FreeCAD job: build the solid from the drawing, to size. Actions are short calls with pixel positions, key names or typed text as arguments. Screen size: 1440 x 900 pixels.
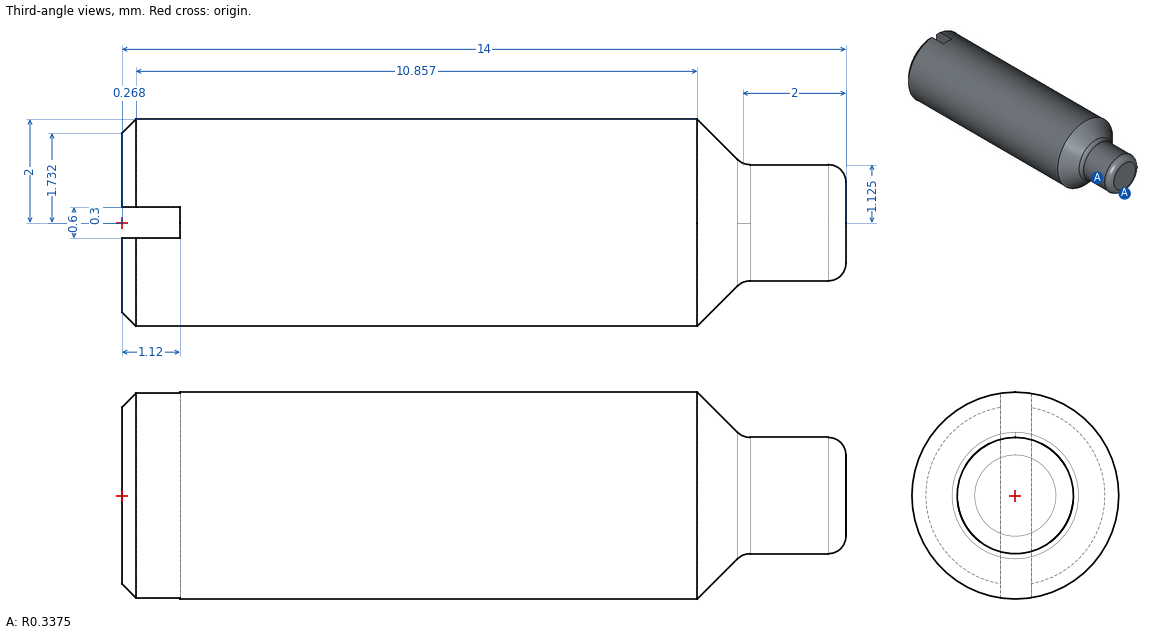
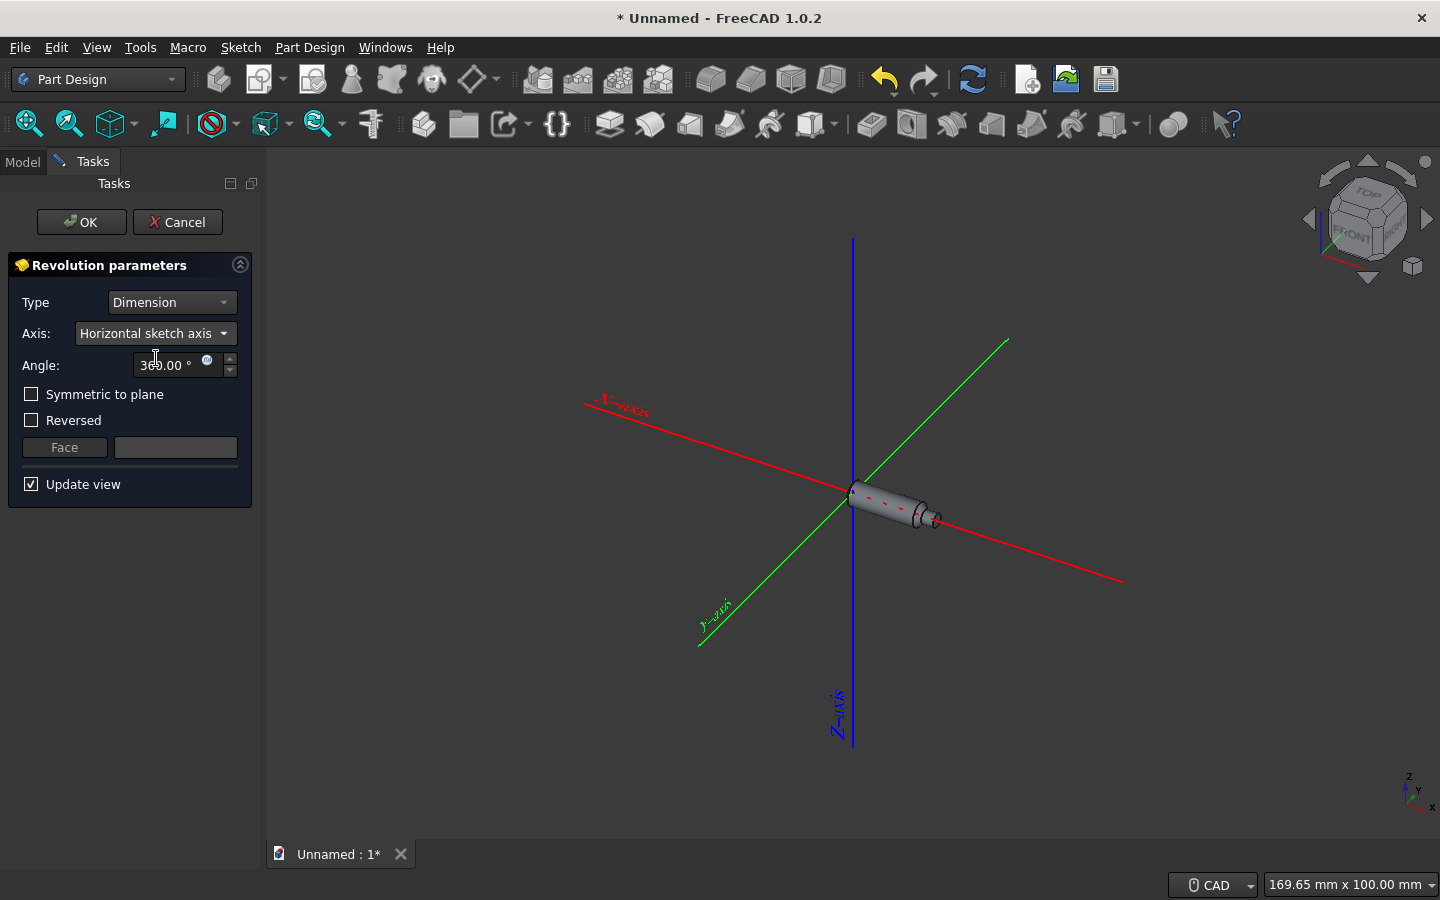
click(82, 222)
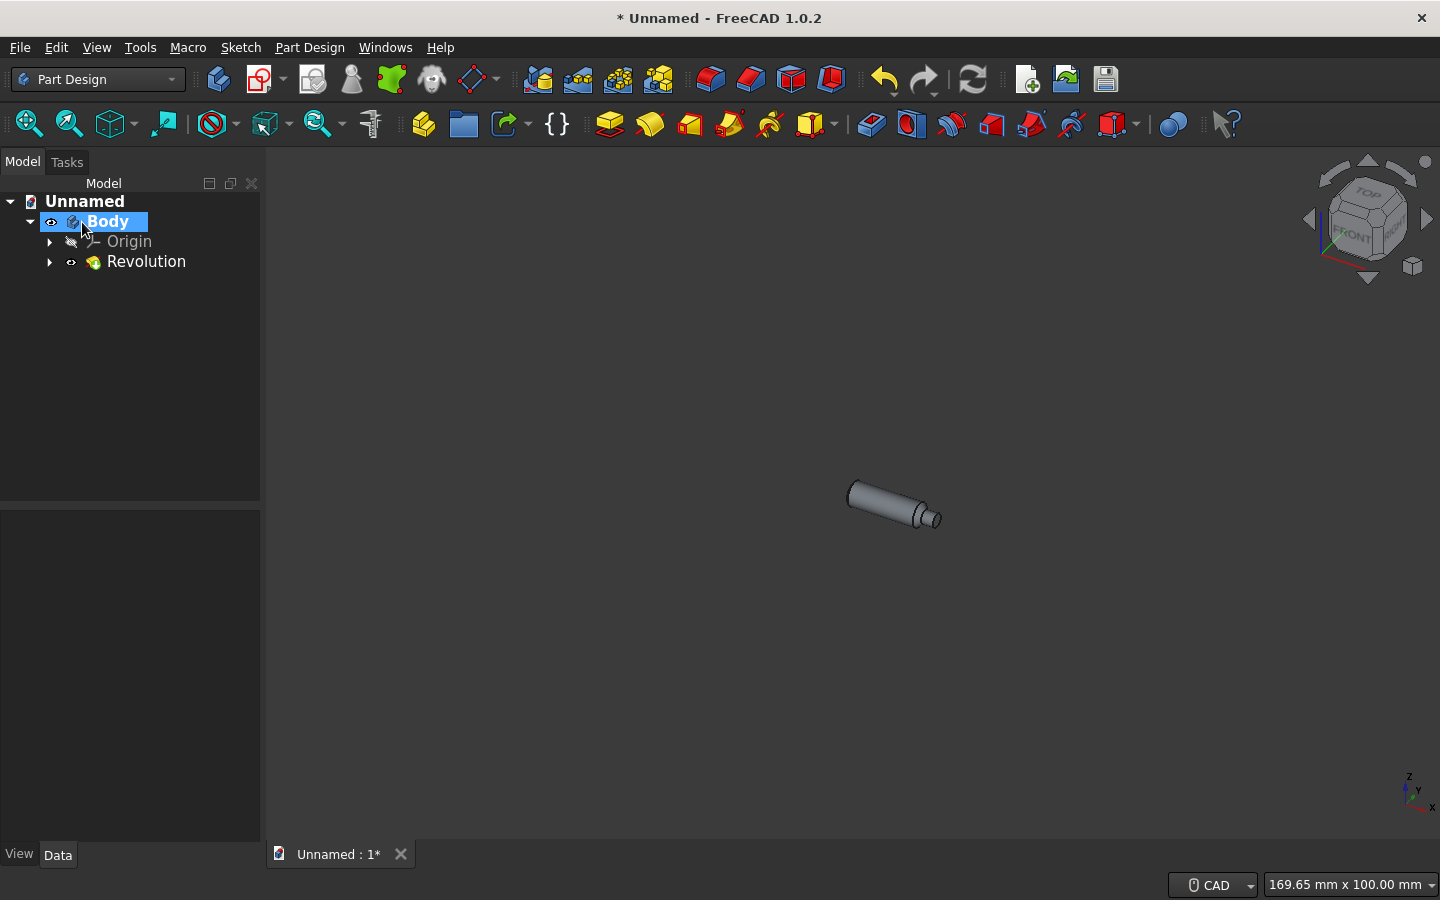
key(v)
key(f)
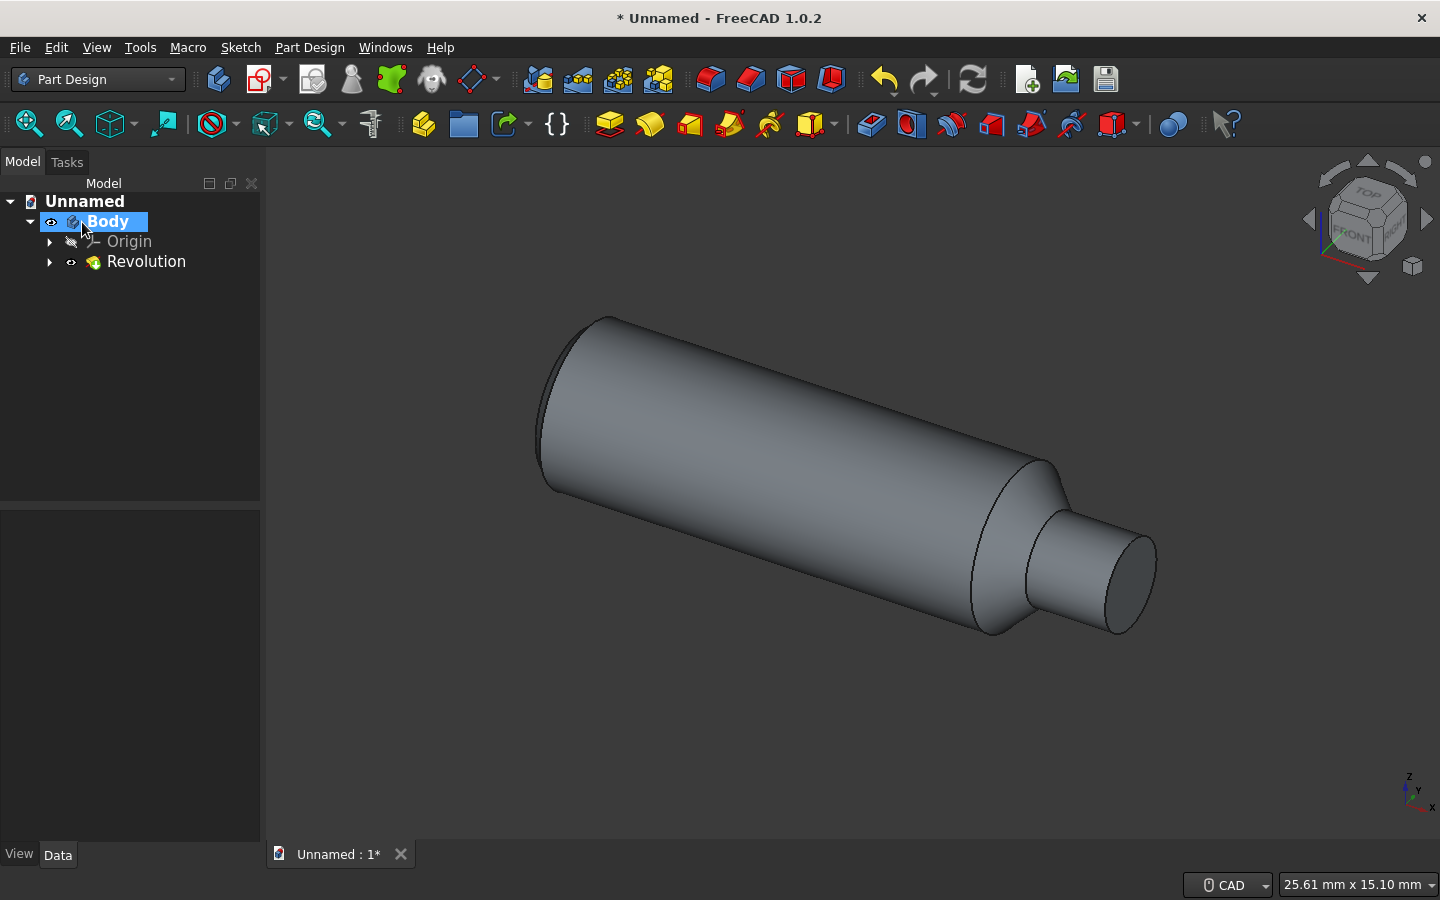
click(260, 80)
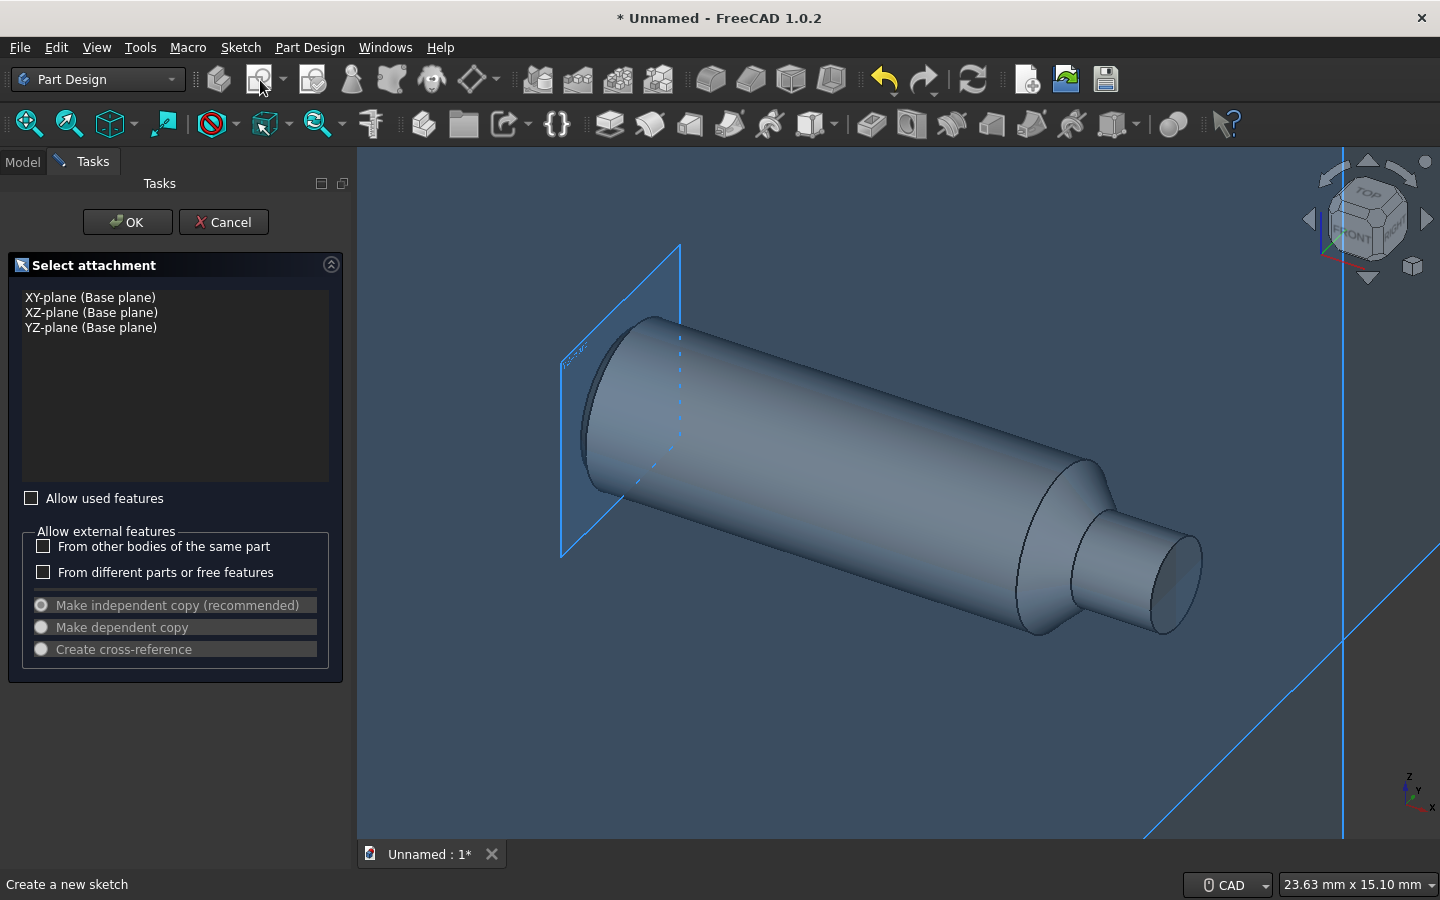
click(82, 298)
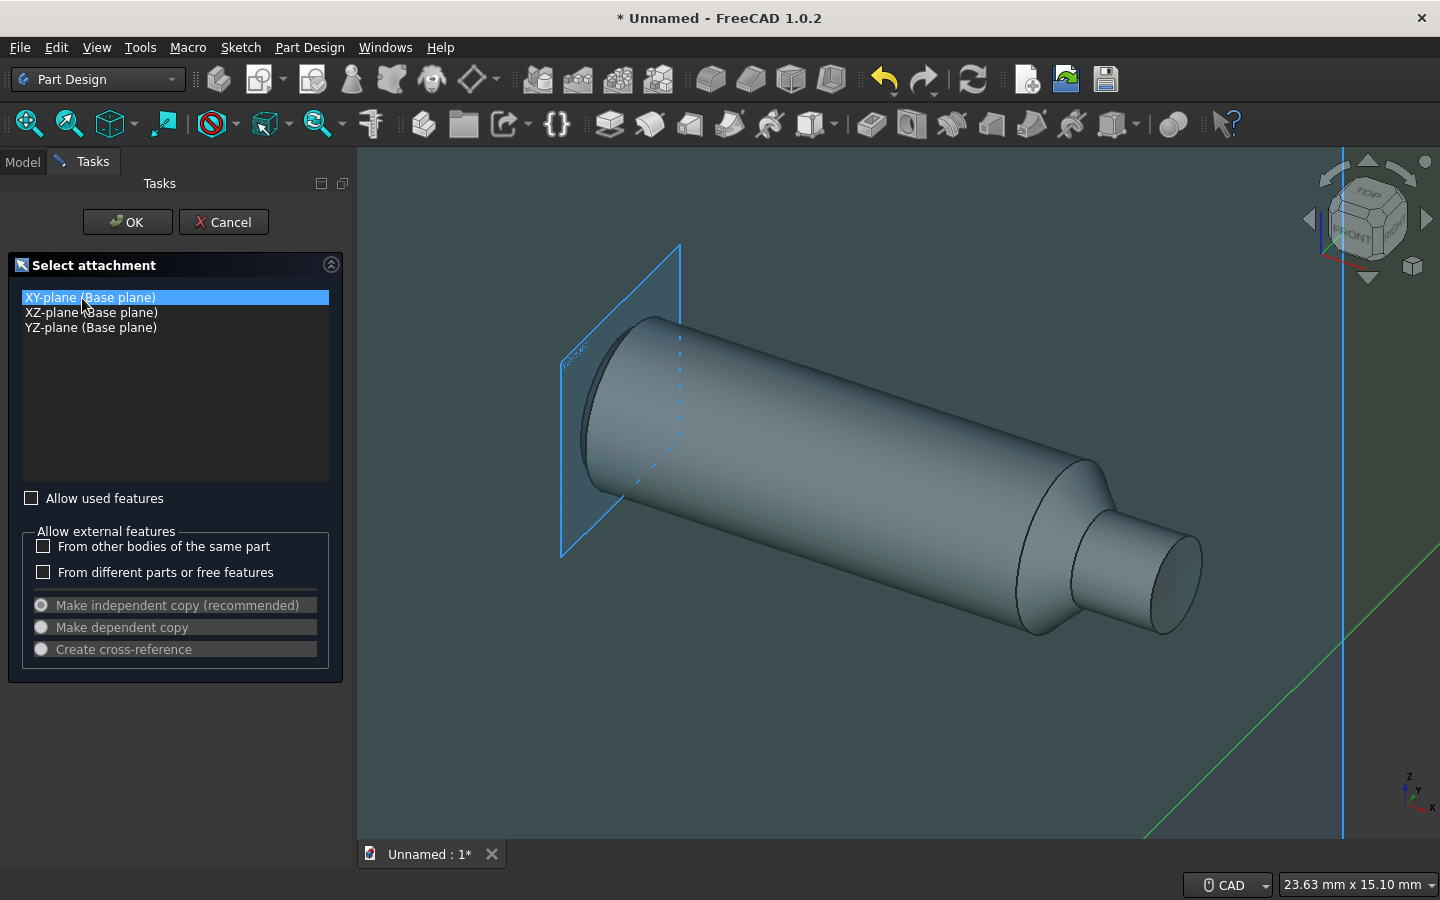
click(128, 222)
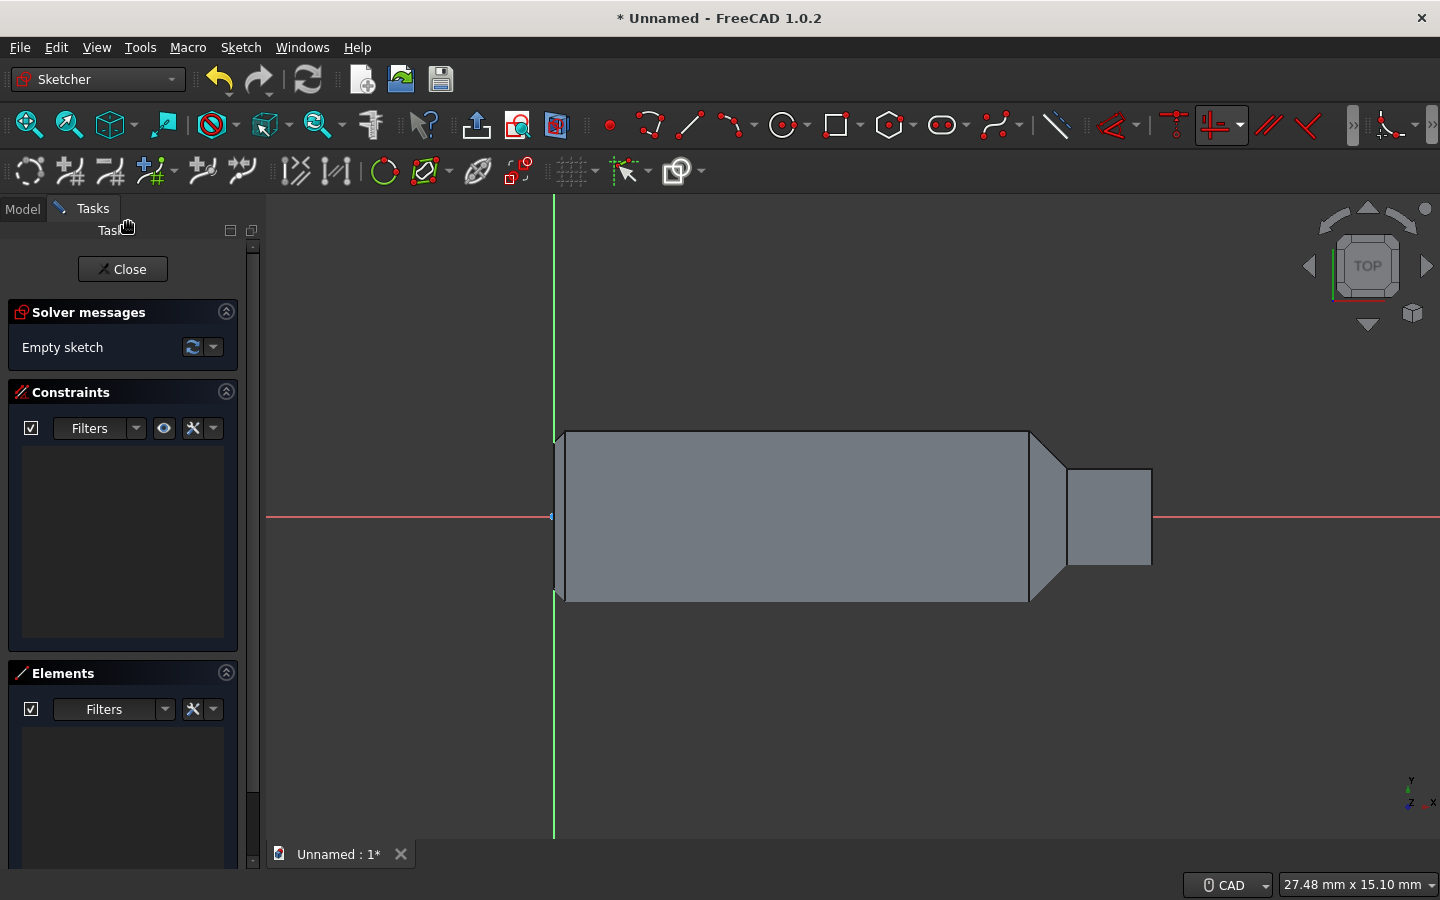
key(q)
key(s)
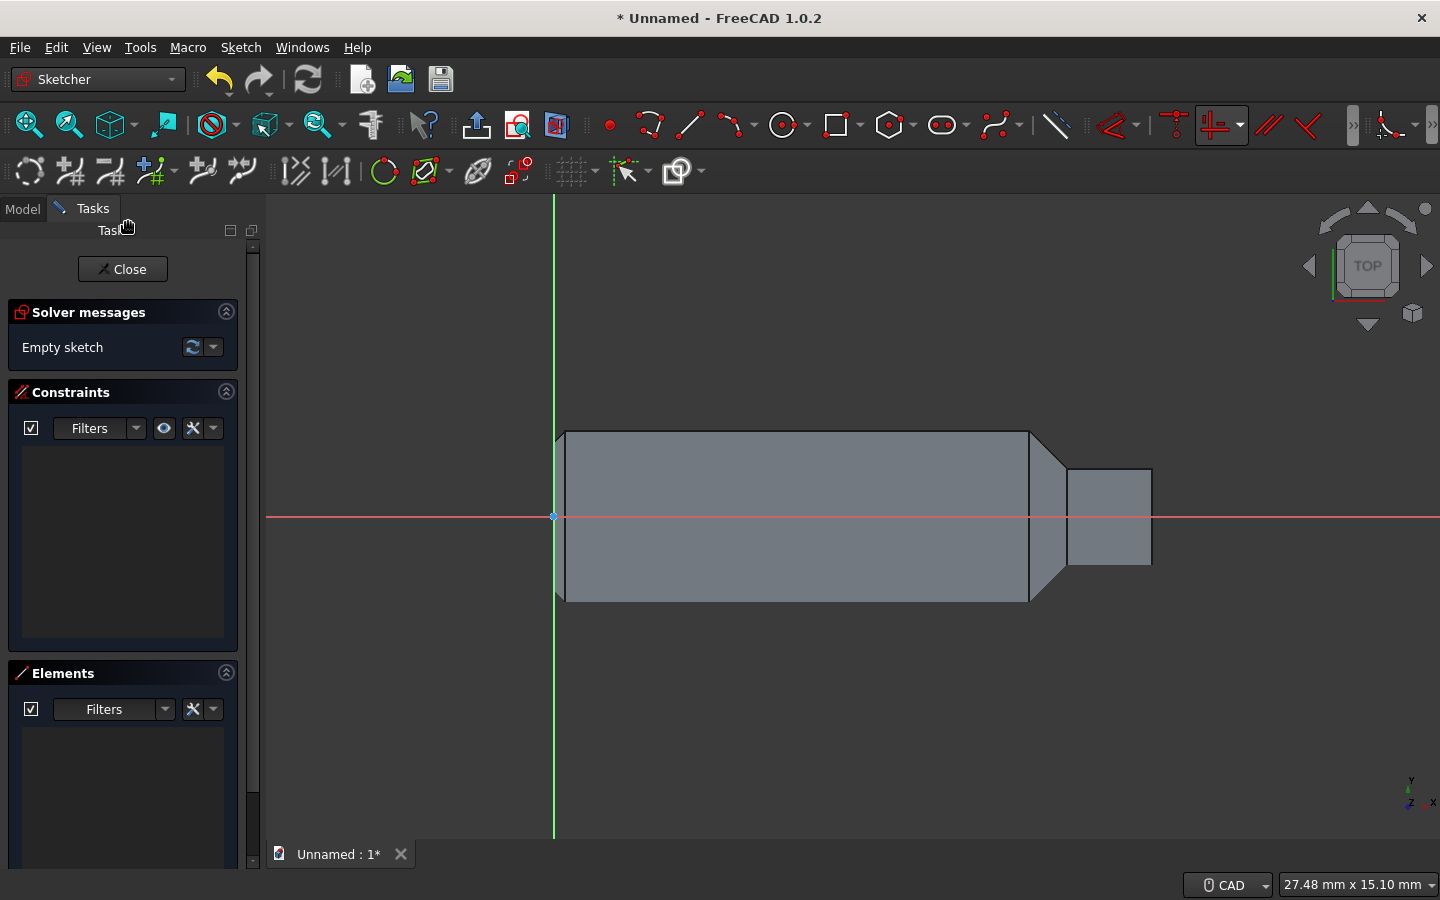
scroll(561, 517, up, 13)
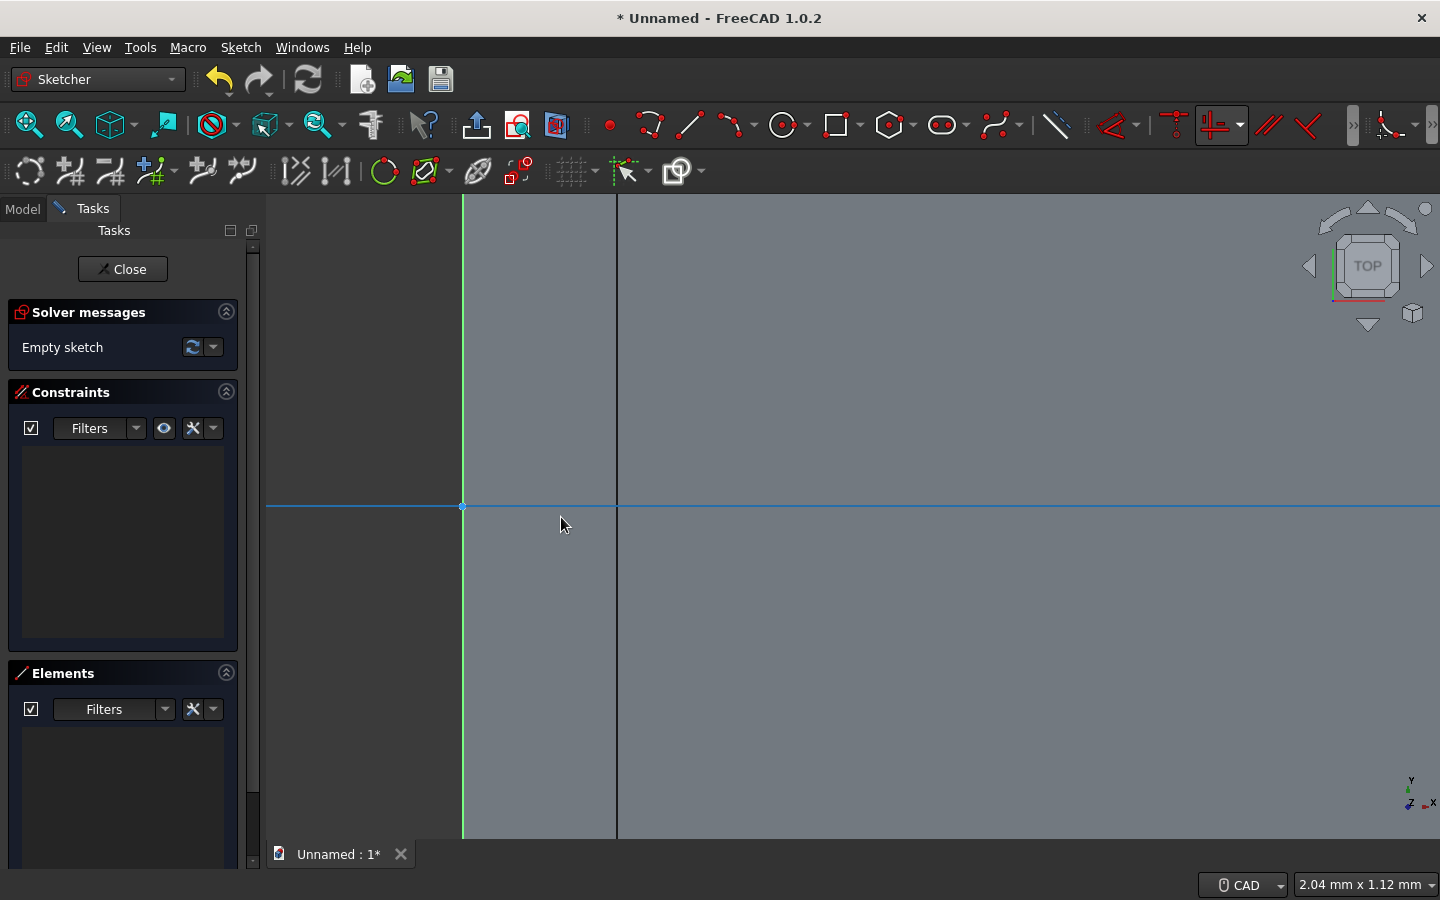
click(836, 126)